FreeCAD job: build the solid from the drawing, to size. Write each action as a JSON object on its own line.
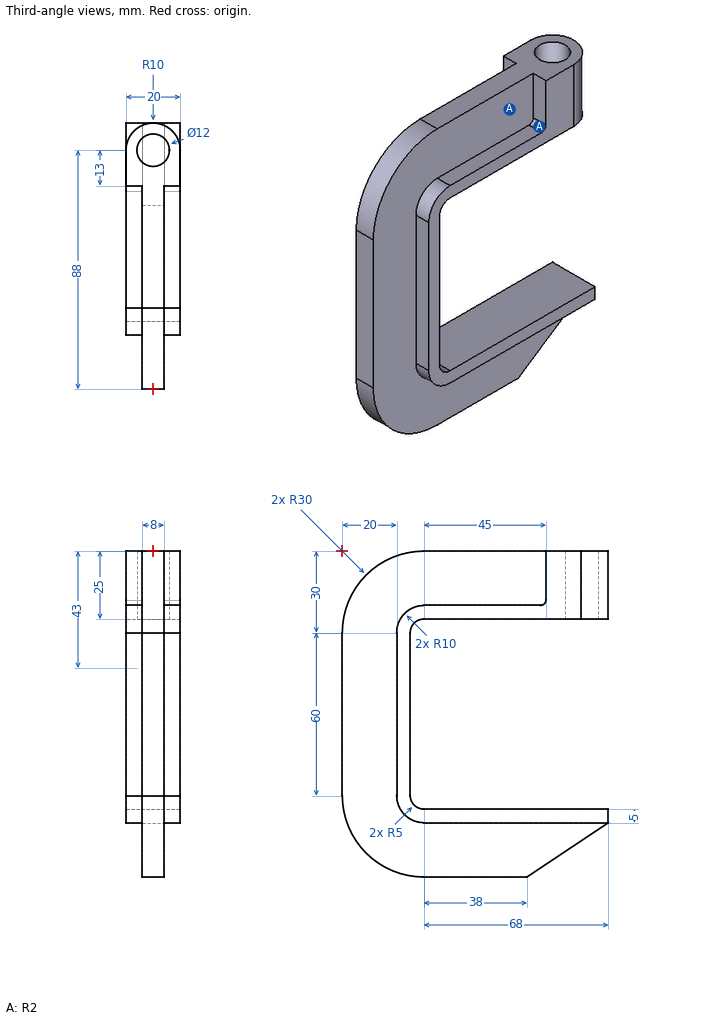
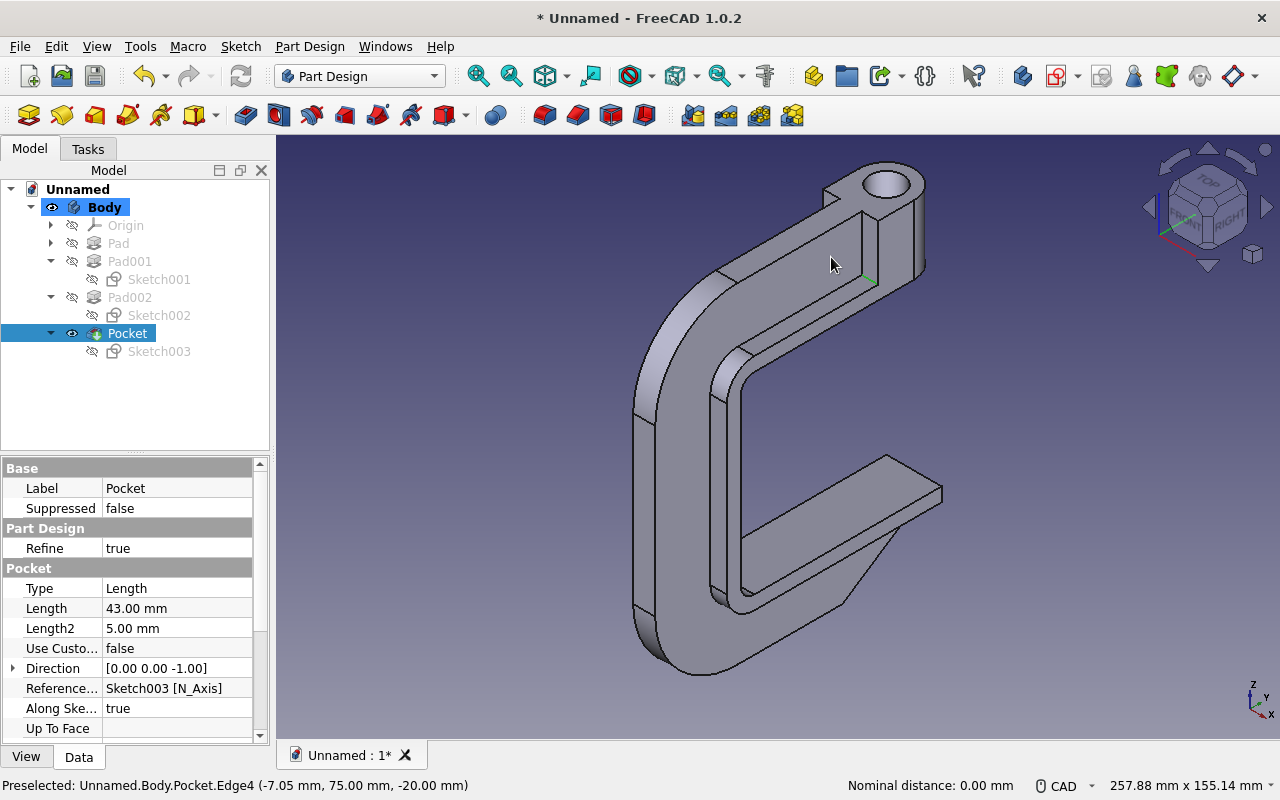
{"action": "left_click", "coordinate": [545, 116]}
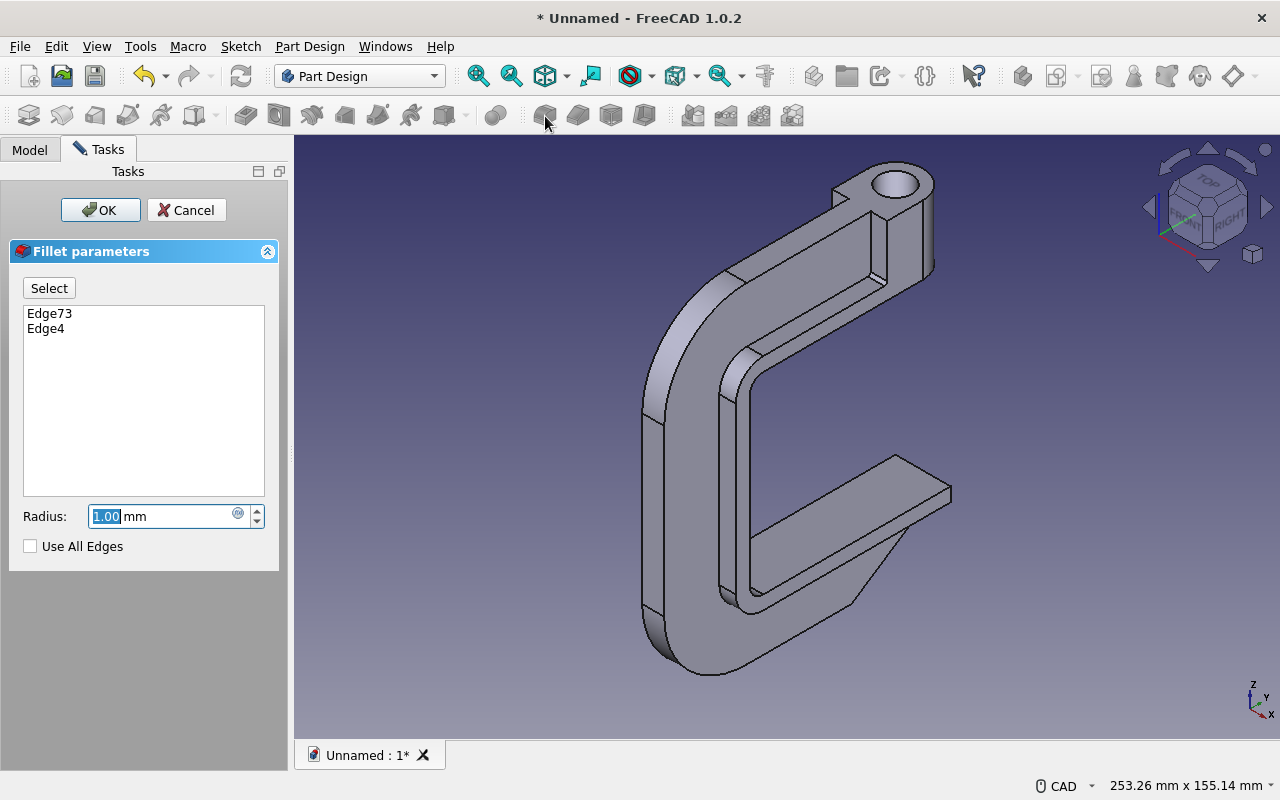
{"action": "type", "text": "2"}
{"action": "key", "text": "Tab"}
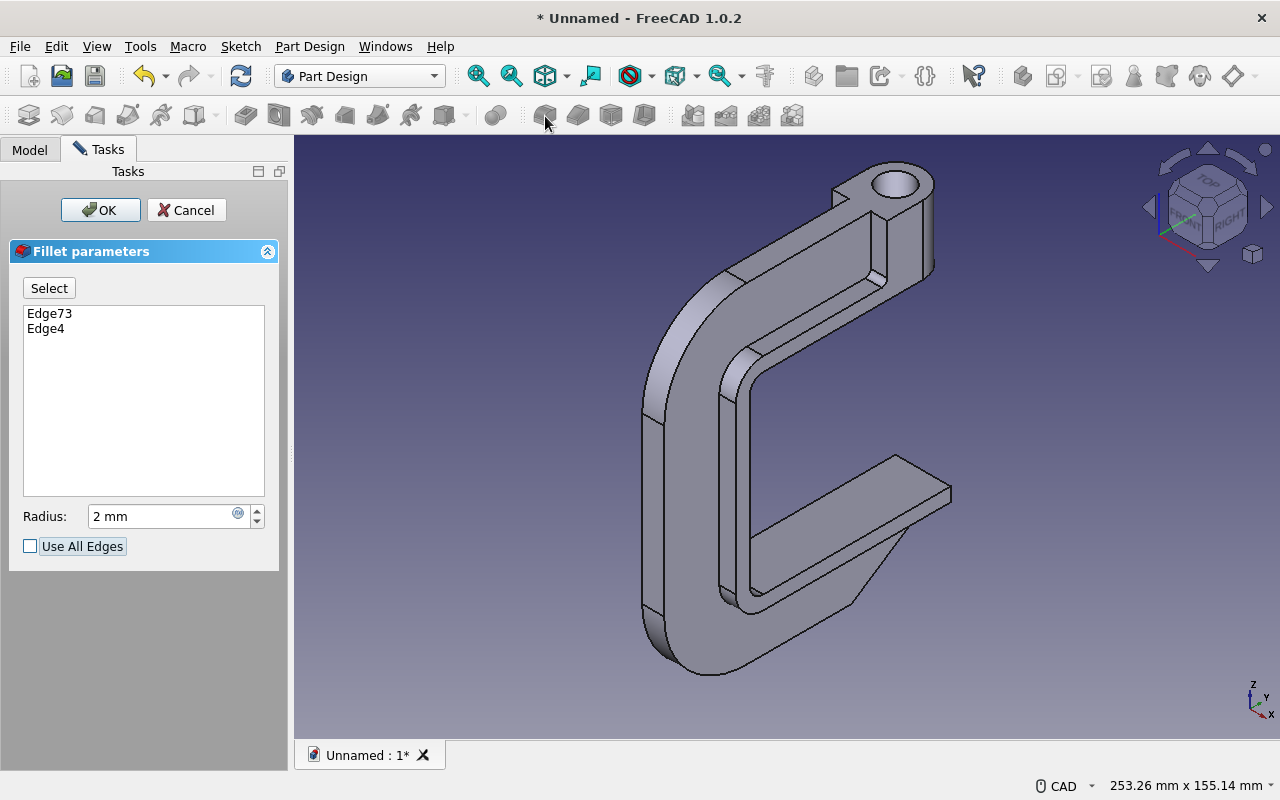
{"action": "left_click", "coordinate": [101, 210]}